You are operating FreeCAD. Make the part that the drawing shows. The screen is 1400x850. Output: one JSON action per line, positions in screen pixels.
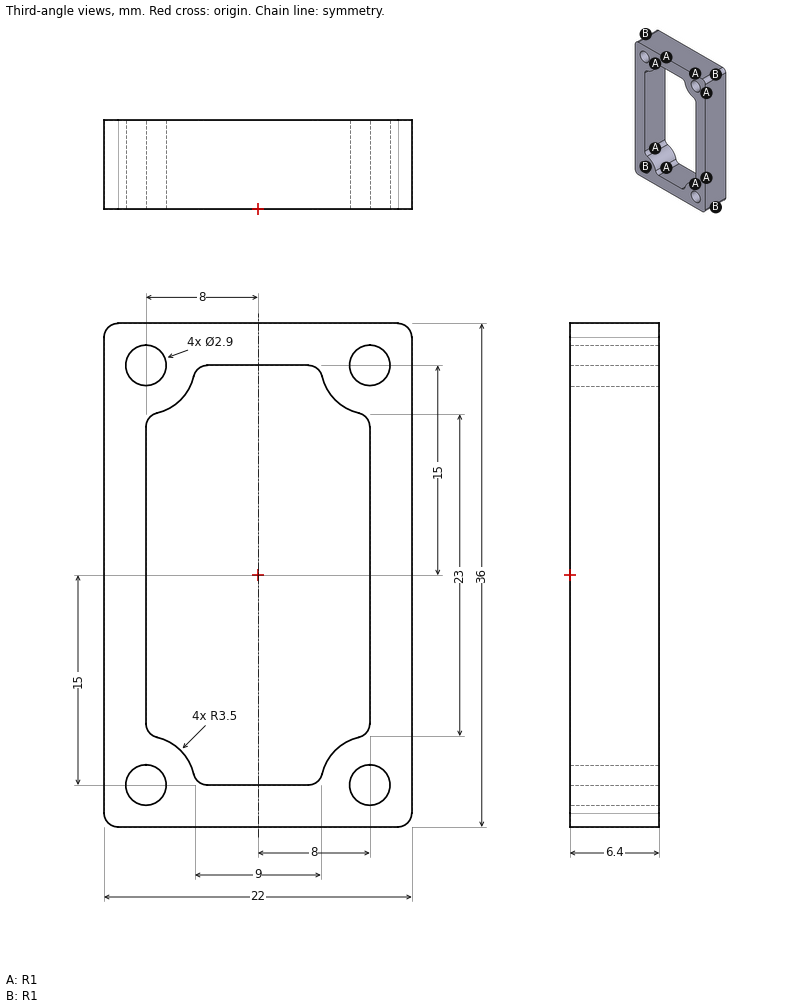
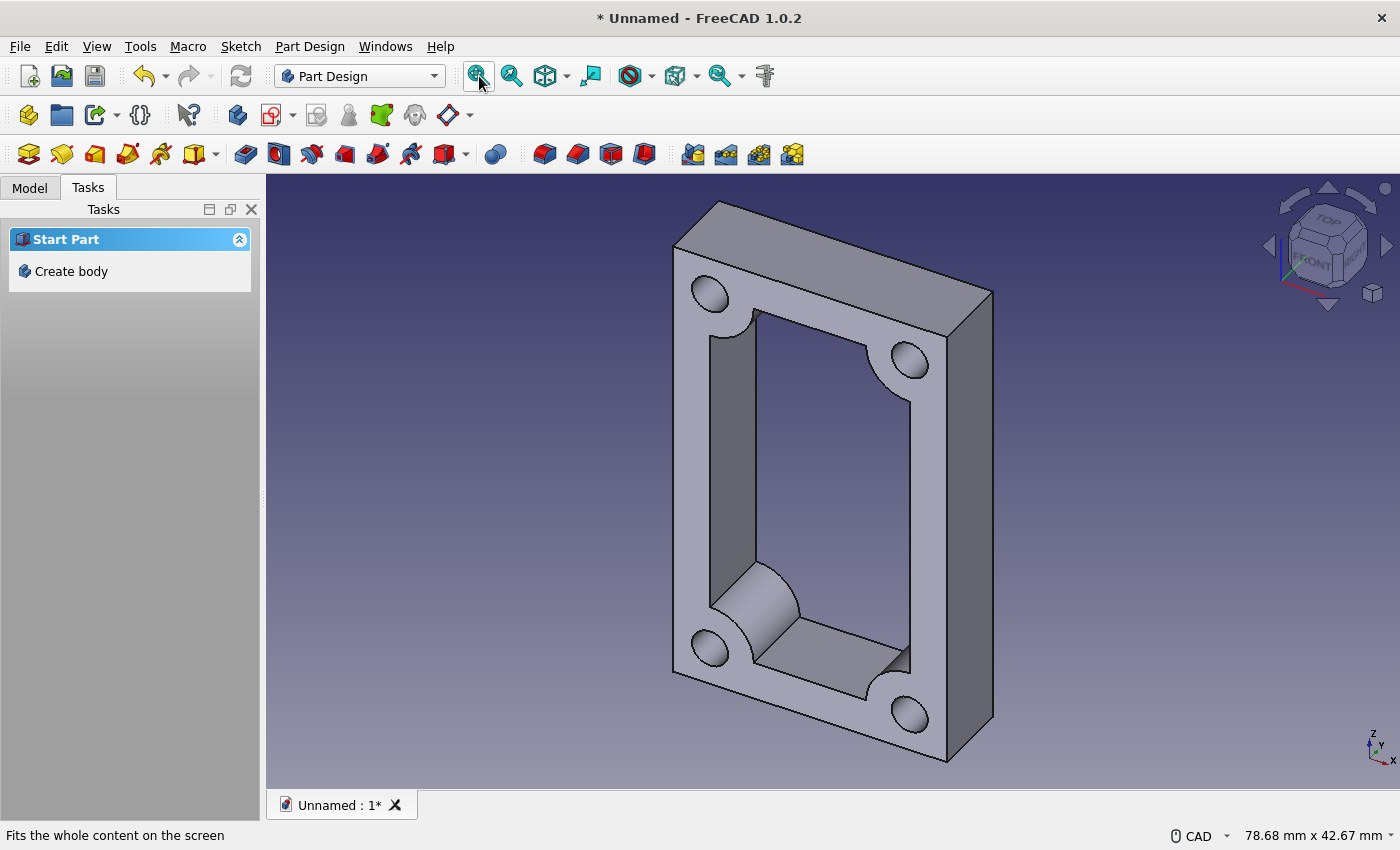
{"action": "key", "text": "0"}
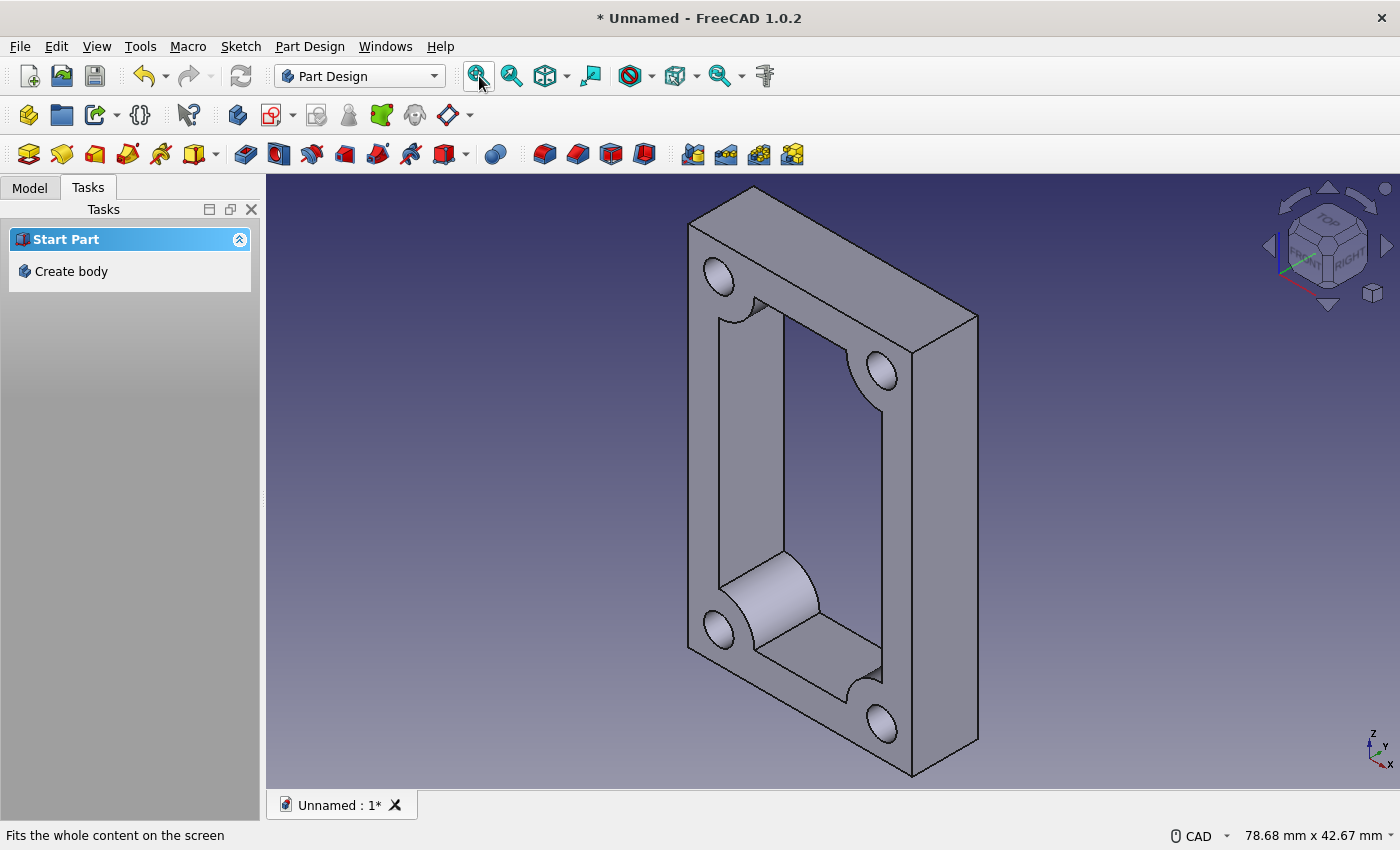
{"action": "key", "text": "2"}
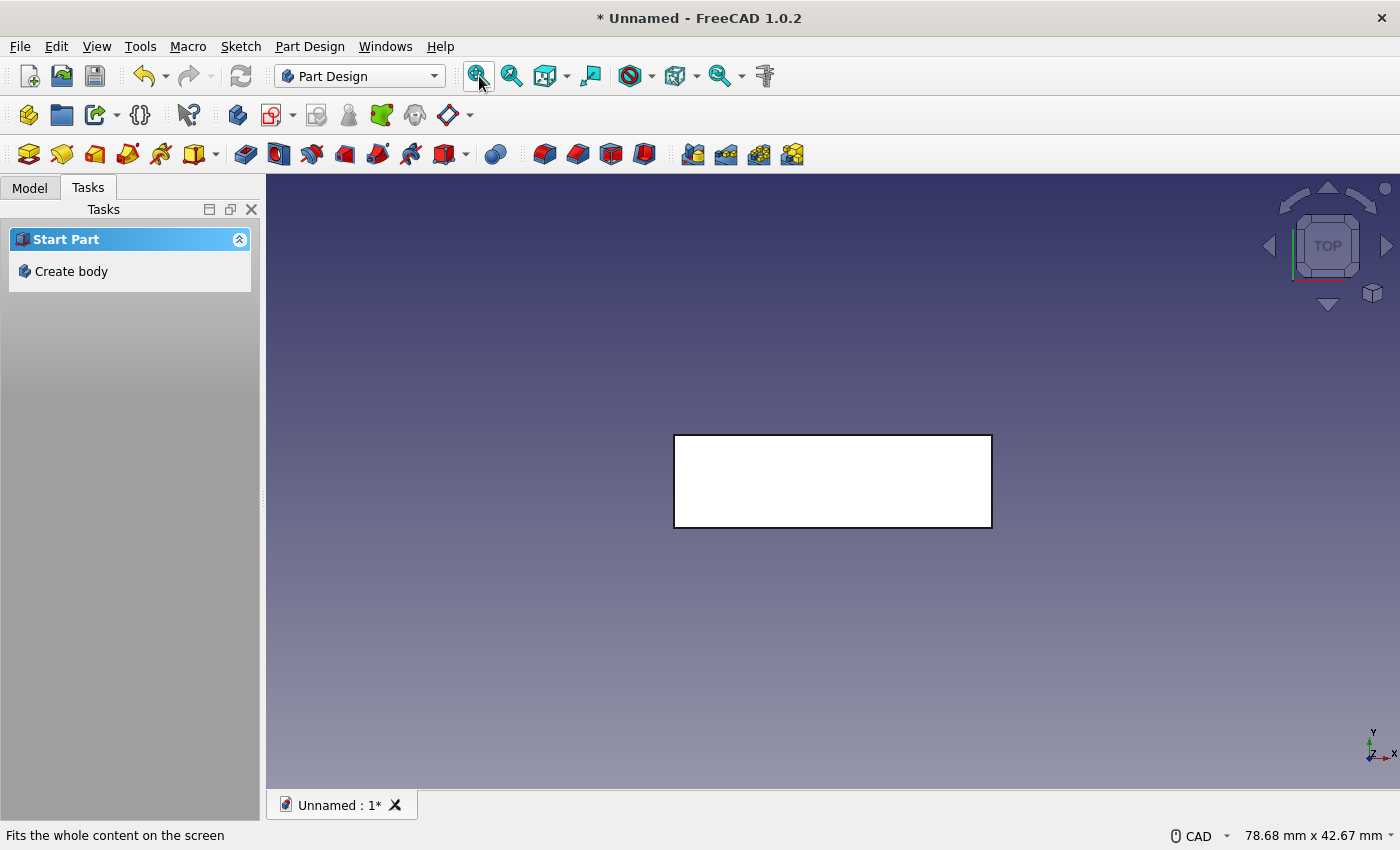
{"action": "left_click", "coordinate": [479, 76]}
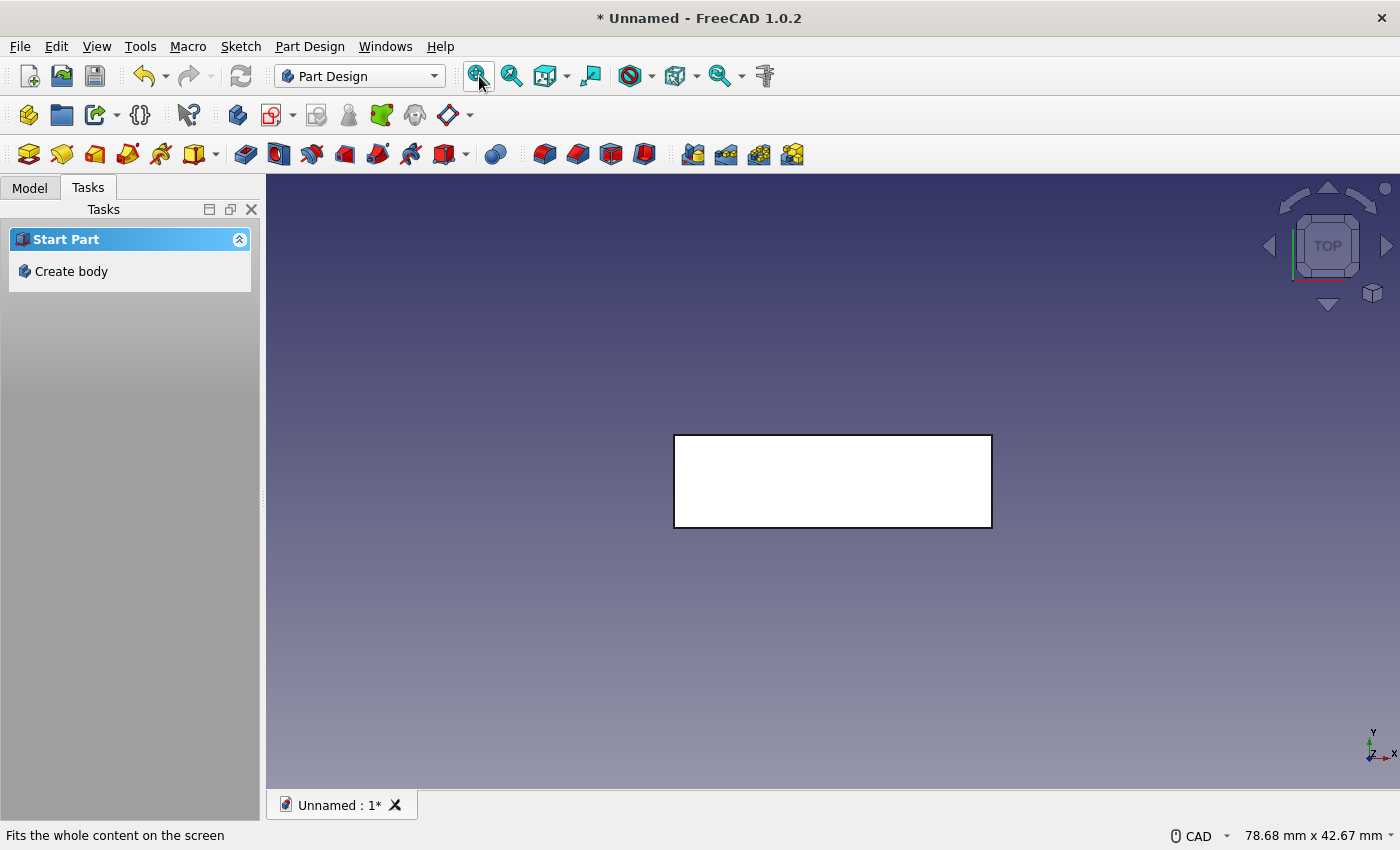
{"action": "key", "text": "1"}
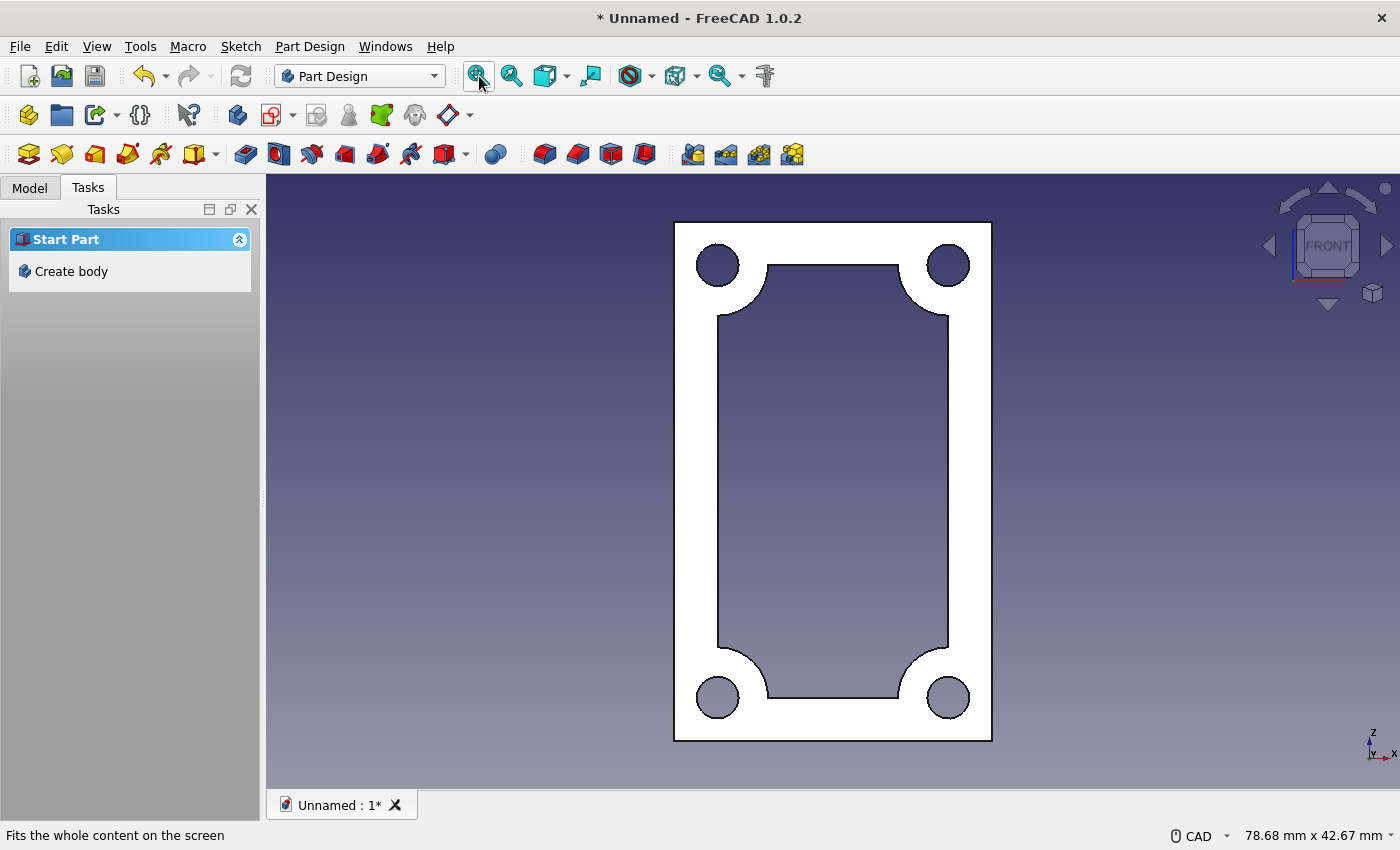
{"action": "key", "text": "3"}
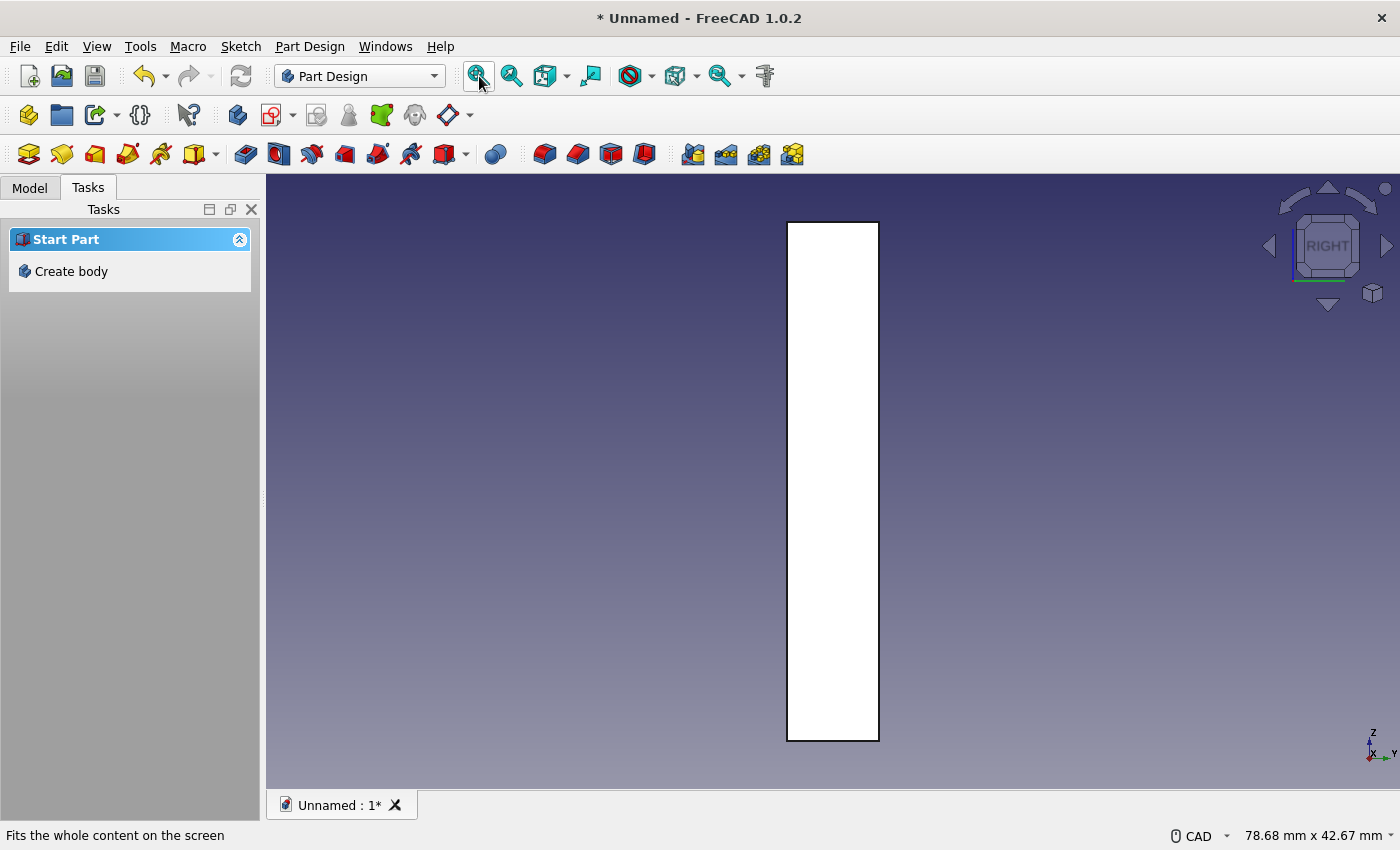
{"action": "key", "text": "5"}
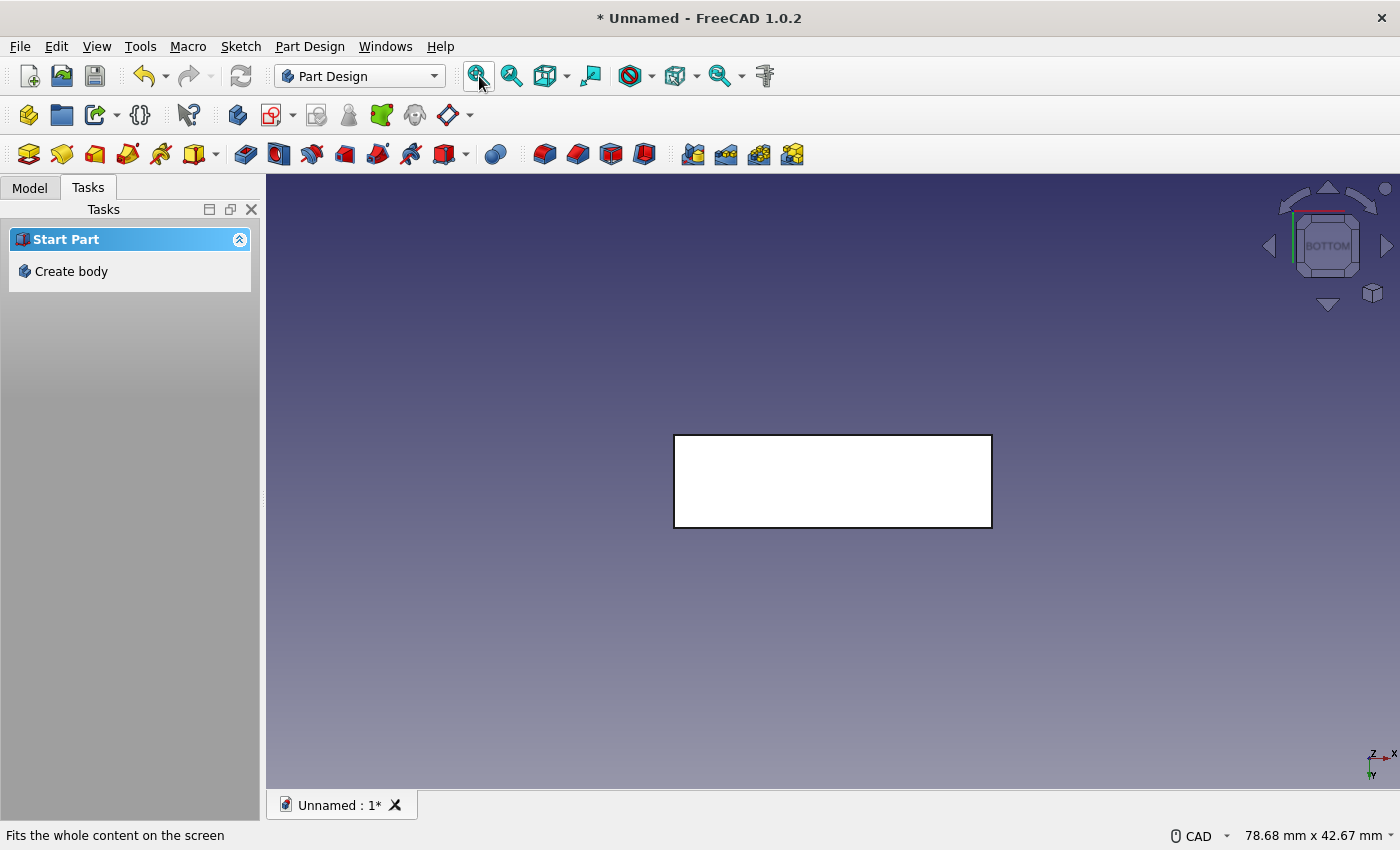
{"action": "left_click", "coordinate": [479, 76]}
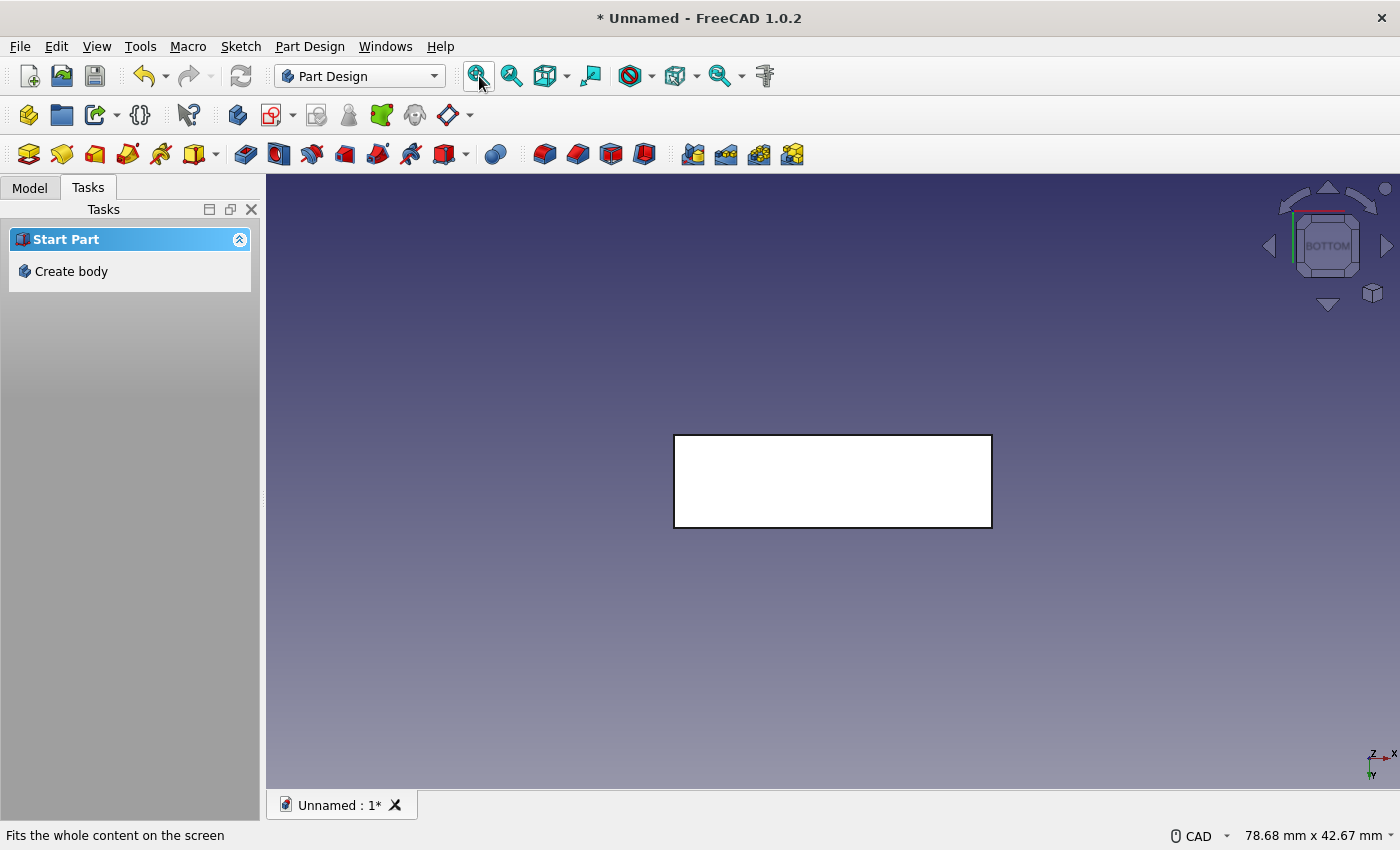
{"action": "key", "text": "4"}